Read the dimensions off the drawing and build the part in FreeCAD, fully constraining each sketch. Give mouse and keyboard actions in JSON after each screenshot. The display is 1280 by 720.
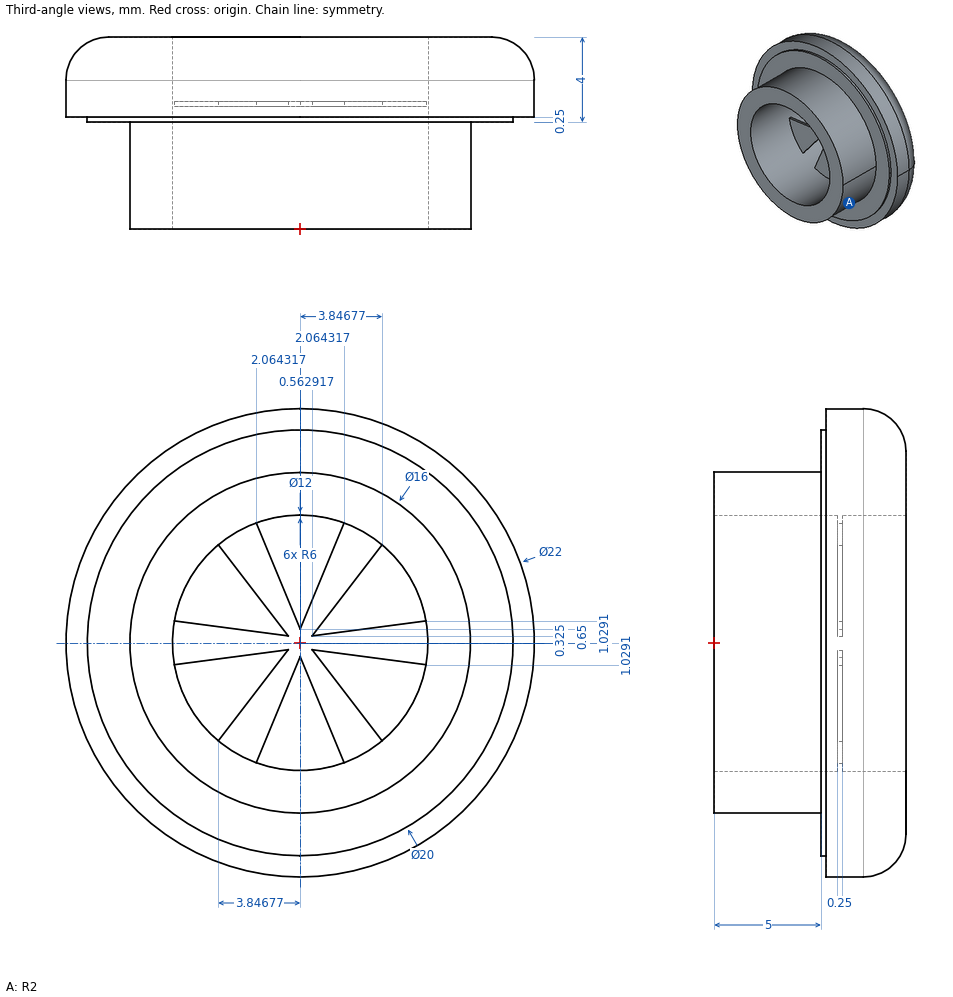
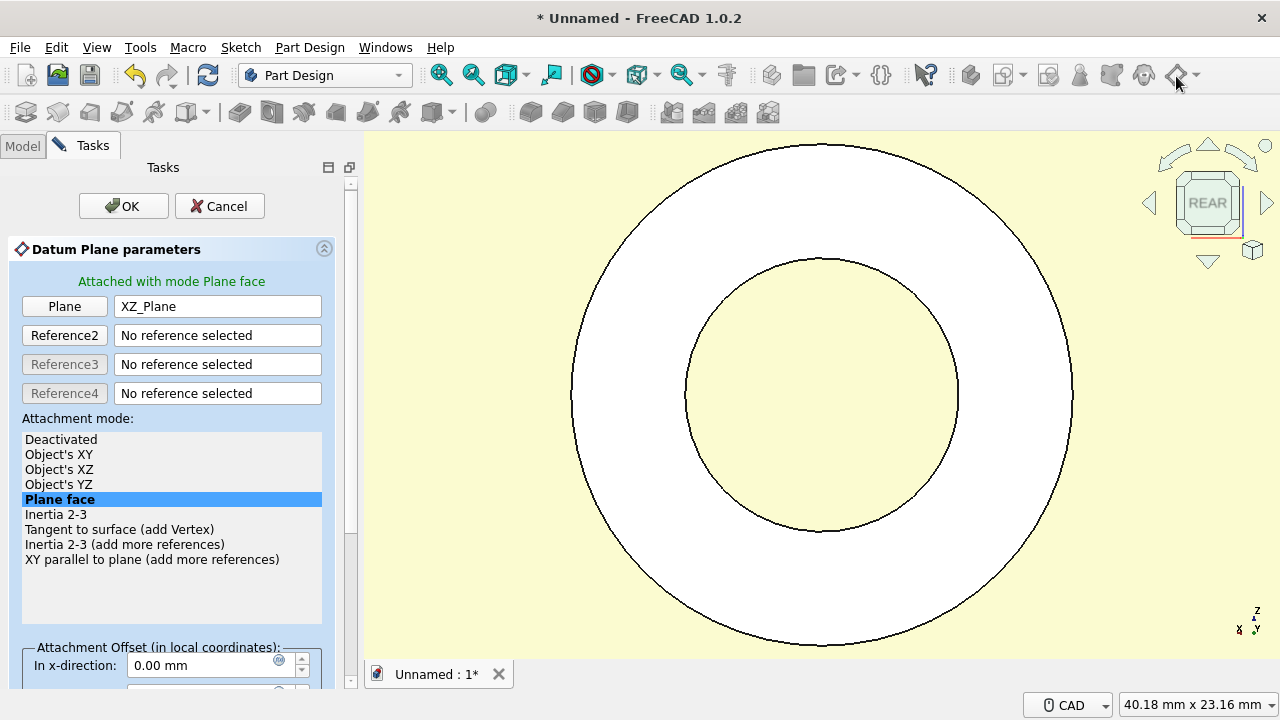
{"action": "scroll", "coordinate": [351, 432], "scroll_direction": "down", "scroll_amount": 2}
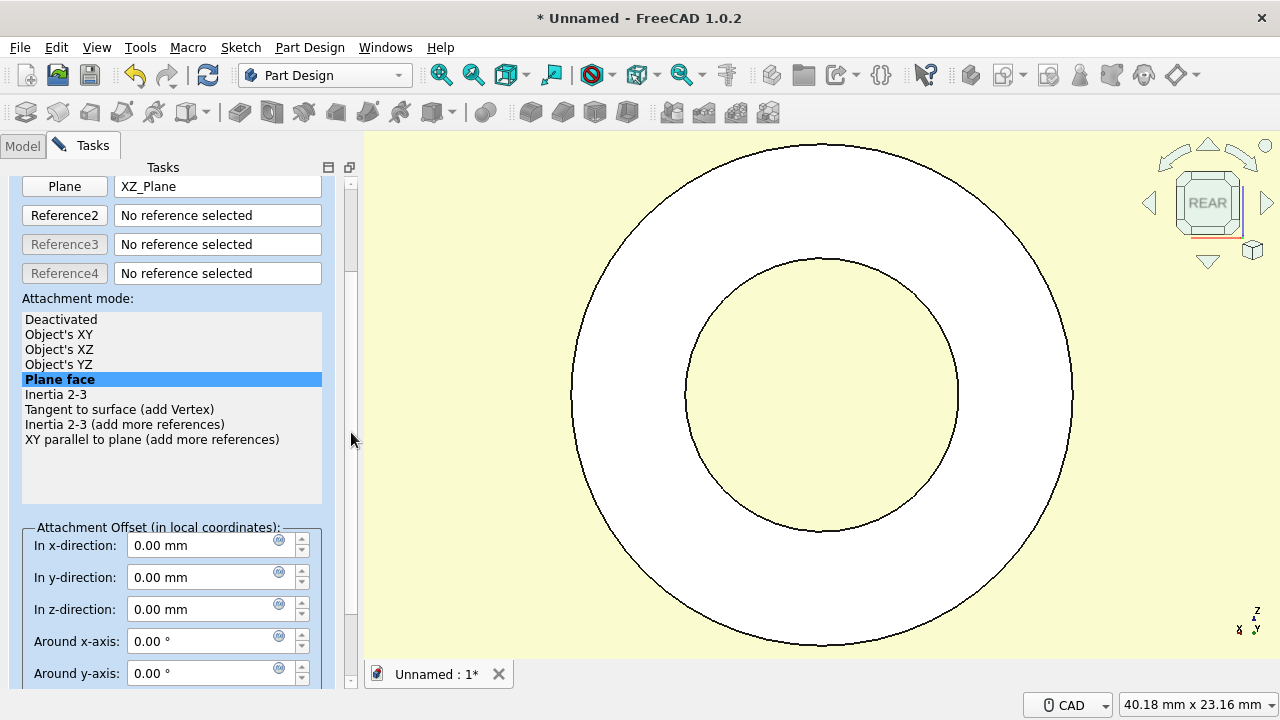
{"action": "triple_click", "coordinate": [210, 609]}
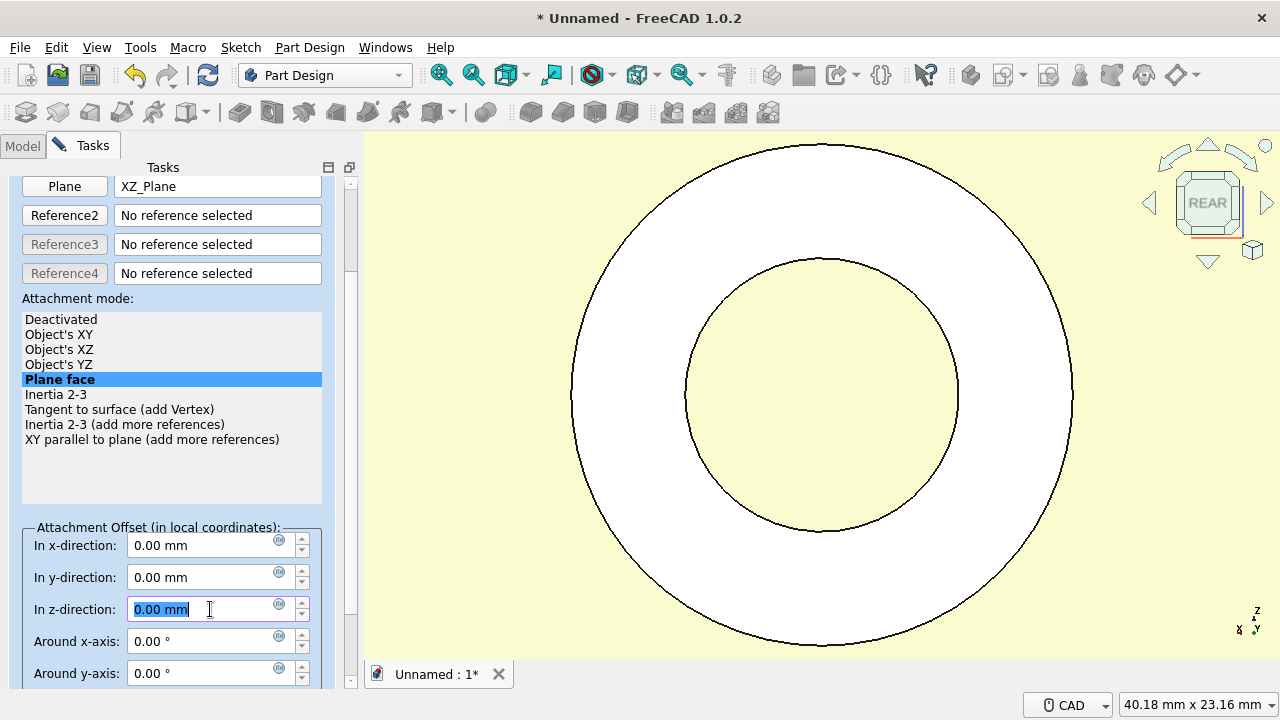
{"action": "type", "text": "-6"}
{"action": "key", "text": "Tab"}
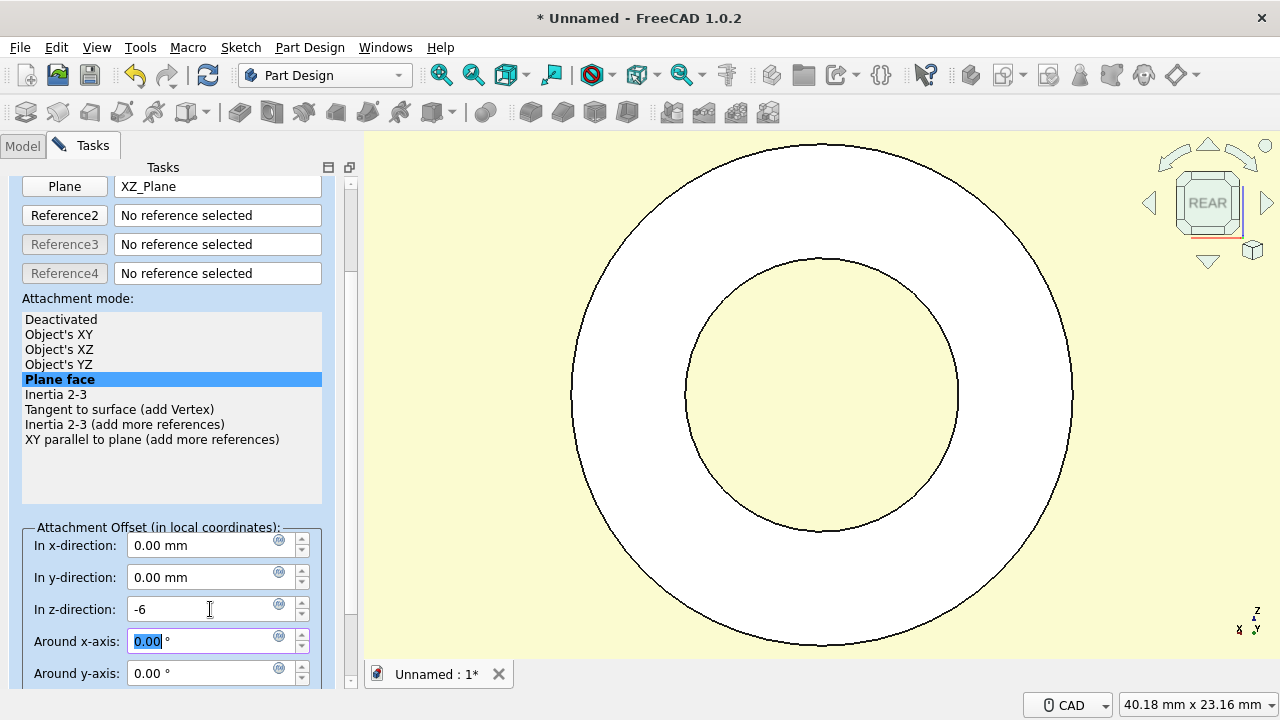
{"action": "scroll", "coordinate": [351, 432], "scroll_direction": "up", "scroll_amount": 3}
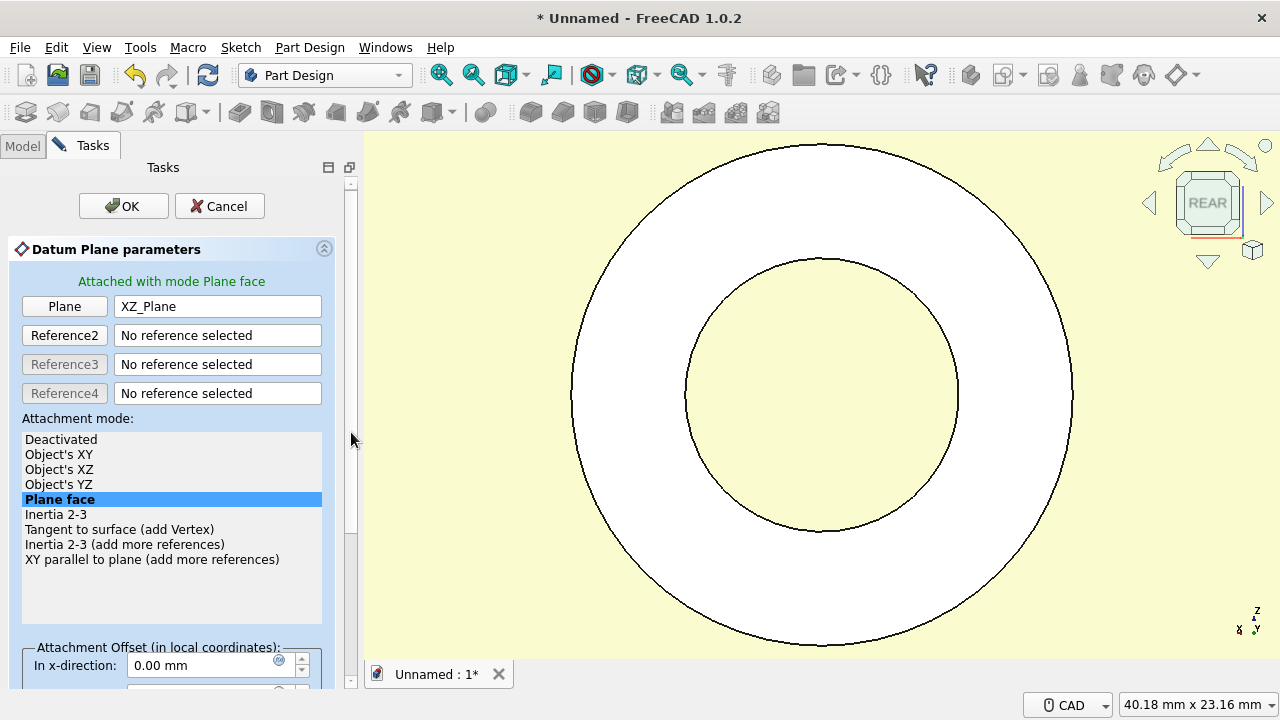
{"action": "left_click", "coordinate": [124, 206]}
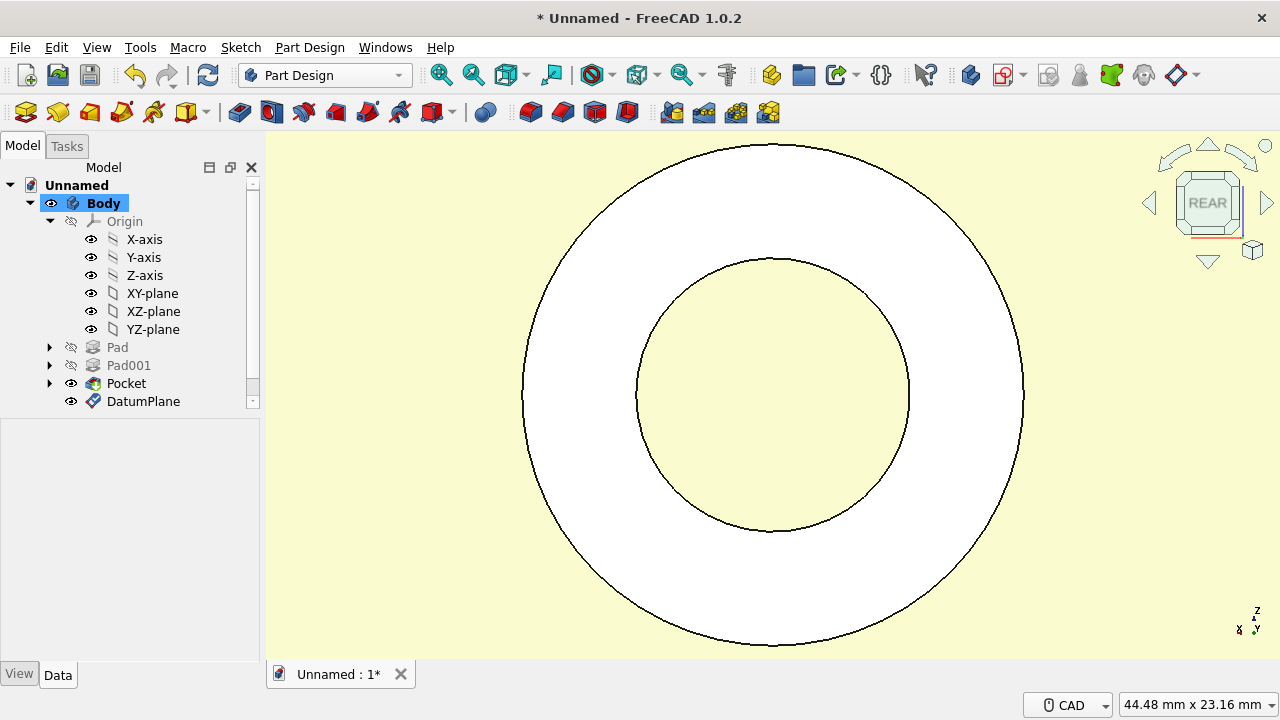
{"action": "left_click", "coordinate": [116, 401]}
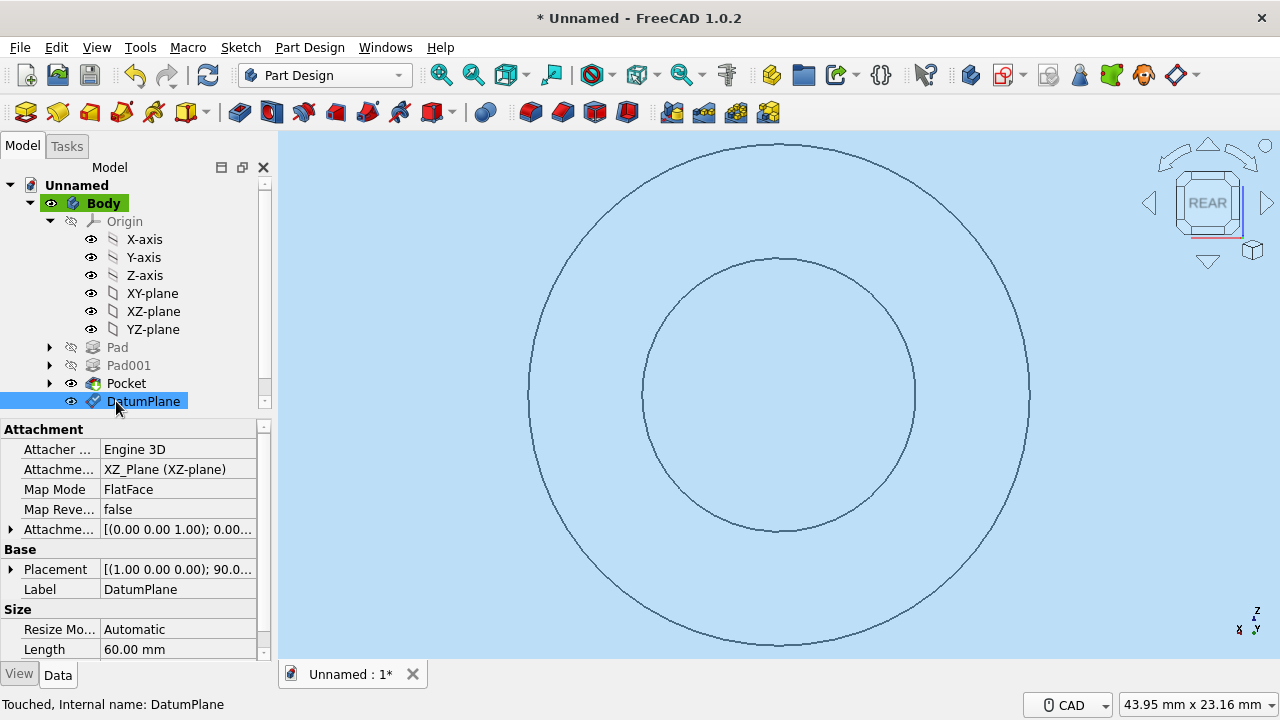
{"action": "left_click", "coordinate": [1004, 76]}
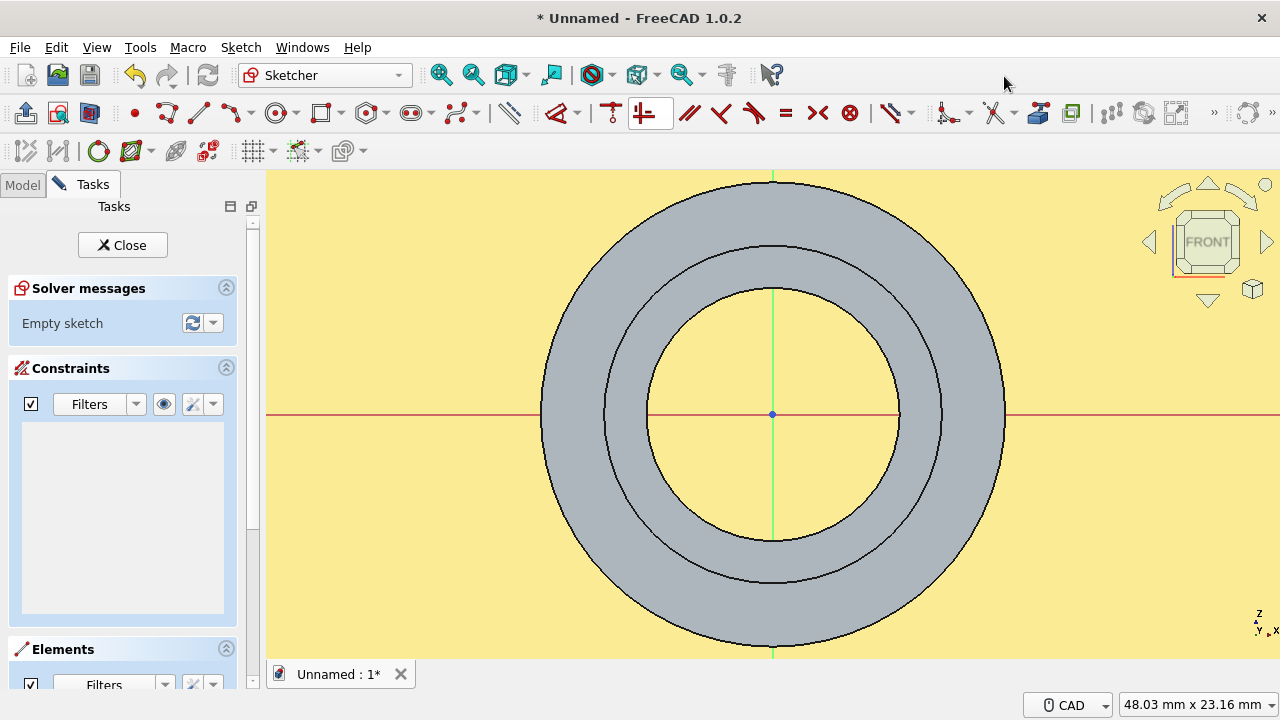
{"action": "key", "text": "q s"}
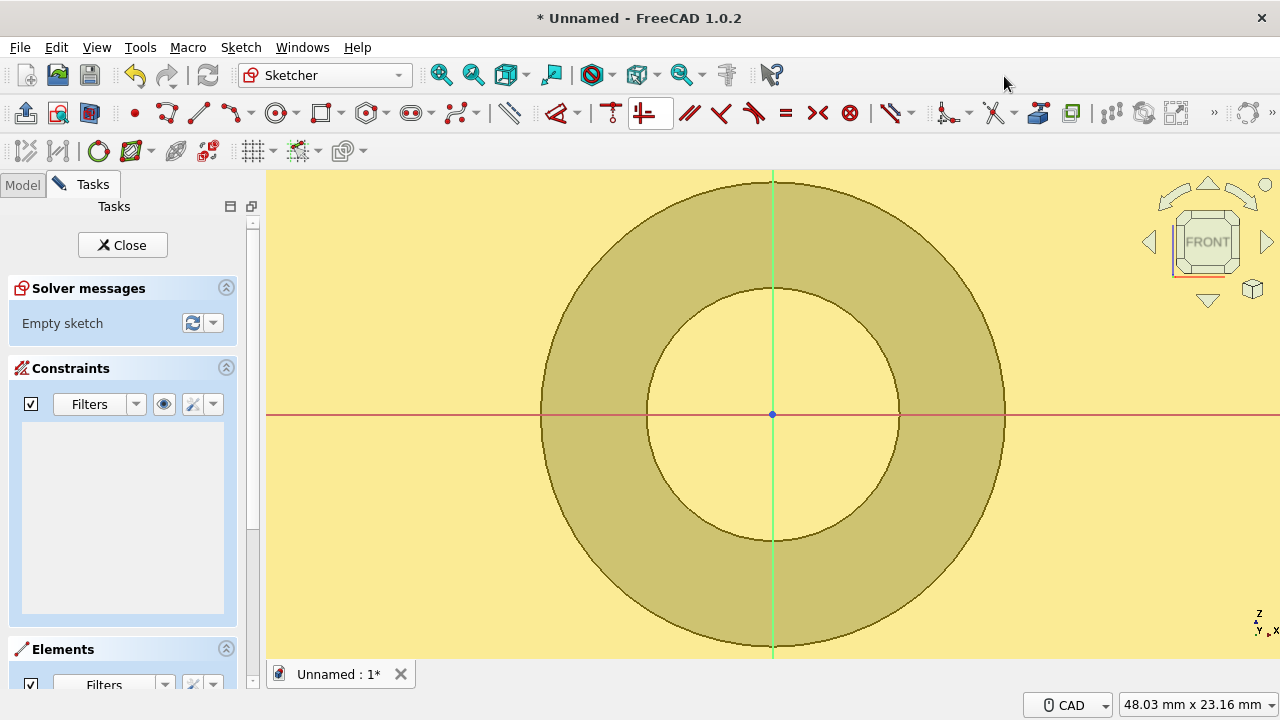
{"action": "left_click", "coordinate": [168, 114]}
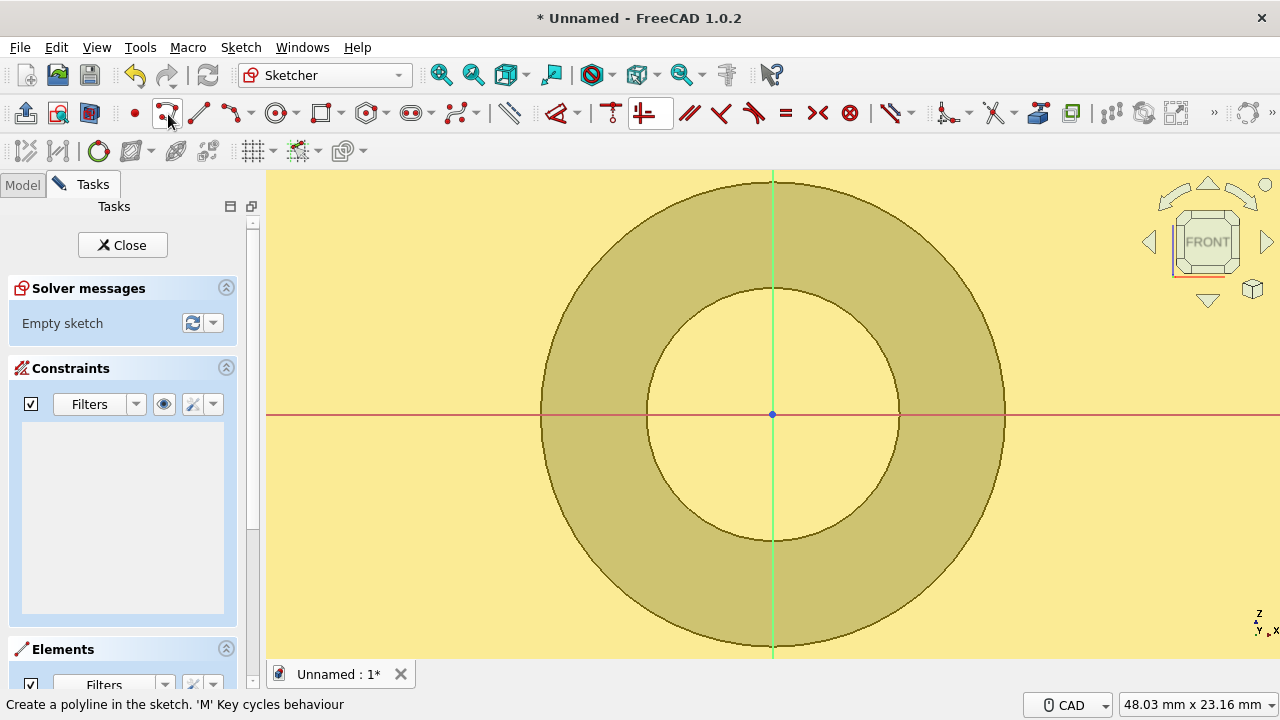
{"action": "left_click", "coordinate": [729, 296]}
{"action": "left_click", "coordinate": [773, 401]}
{"action": "left_click", "coordinate": [817, 296]}
{"action": "right_click", "coordinate": [817, 296]}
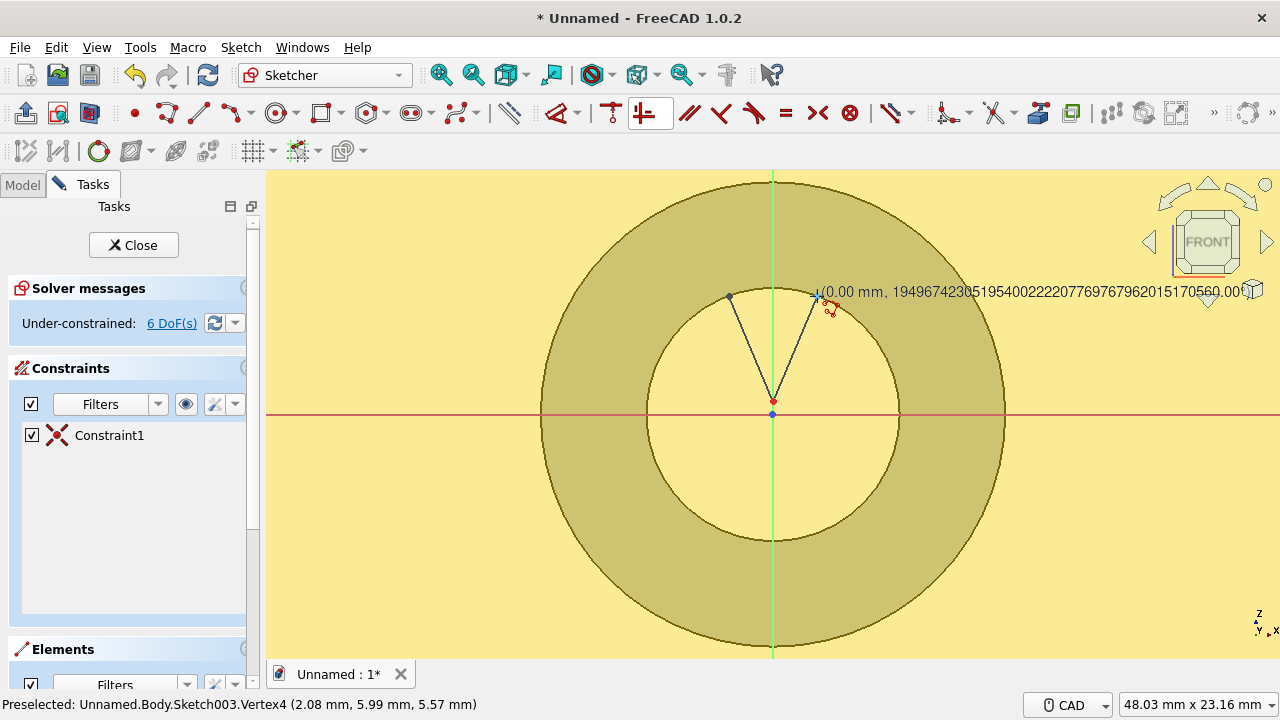
{"action": "key", "text": "g 3 a"}